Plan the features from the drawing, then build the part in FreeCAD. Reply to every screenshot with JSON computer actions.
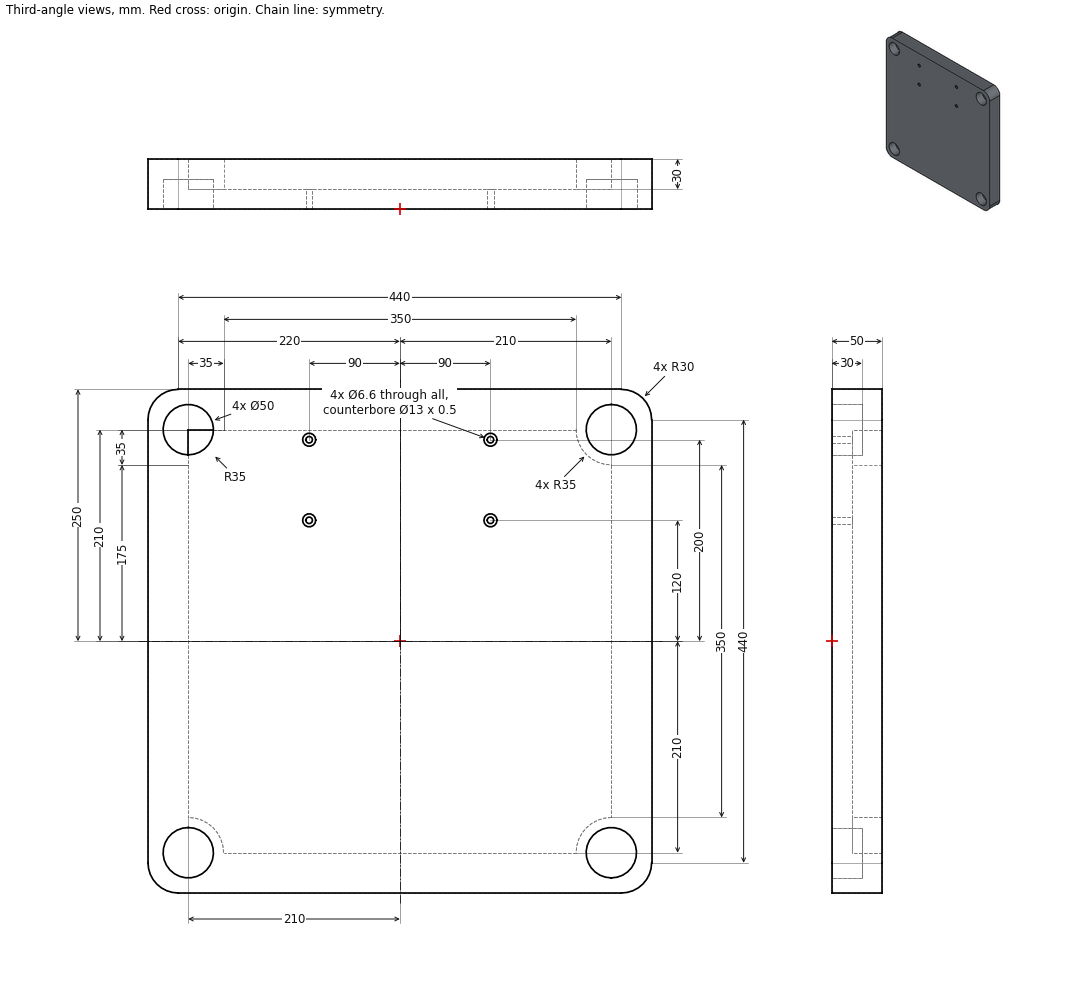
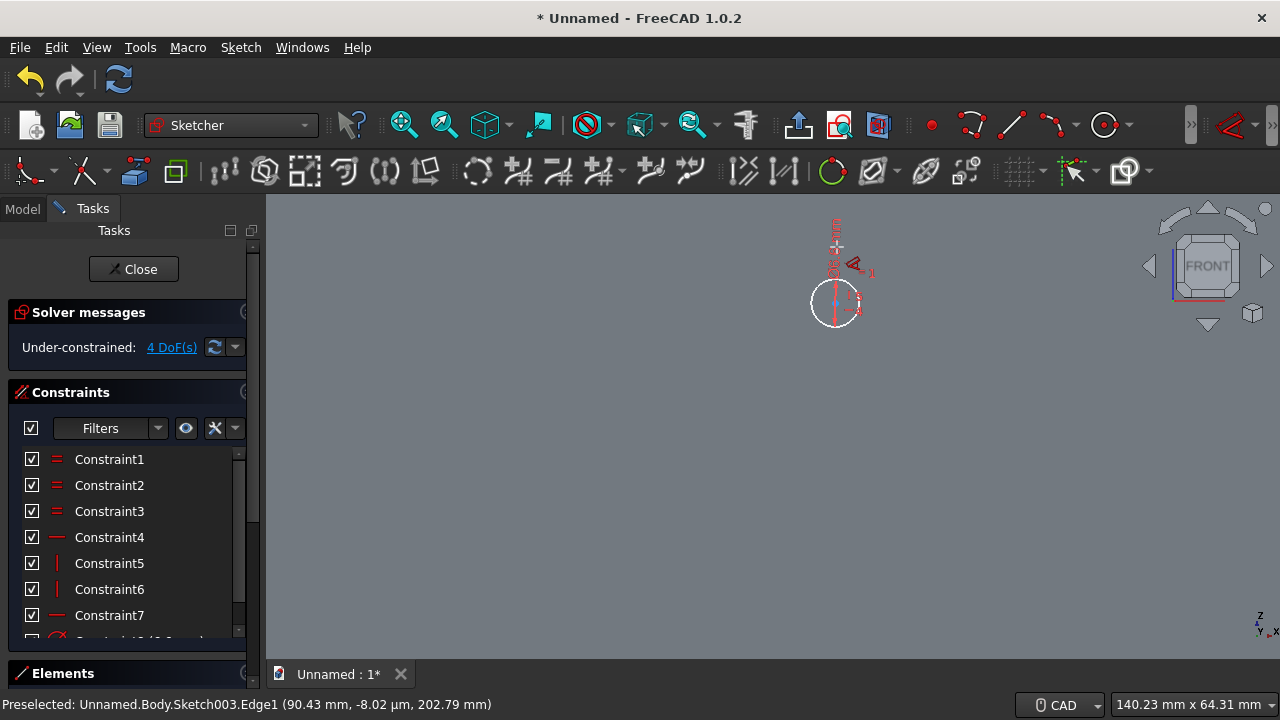
{"action": "scroll", "coordinate": [836, 279], "scroll_direction": "down", "scroll_amount": 8}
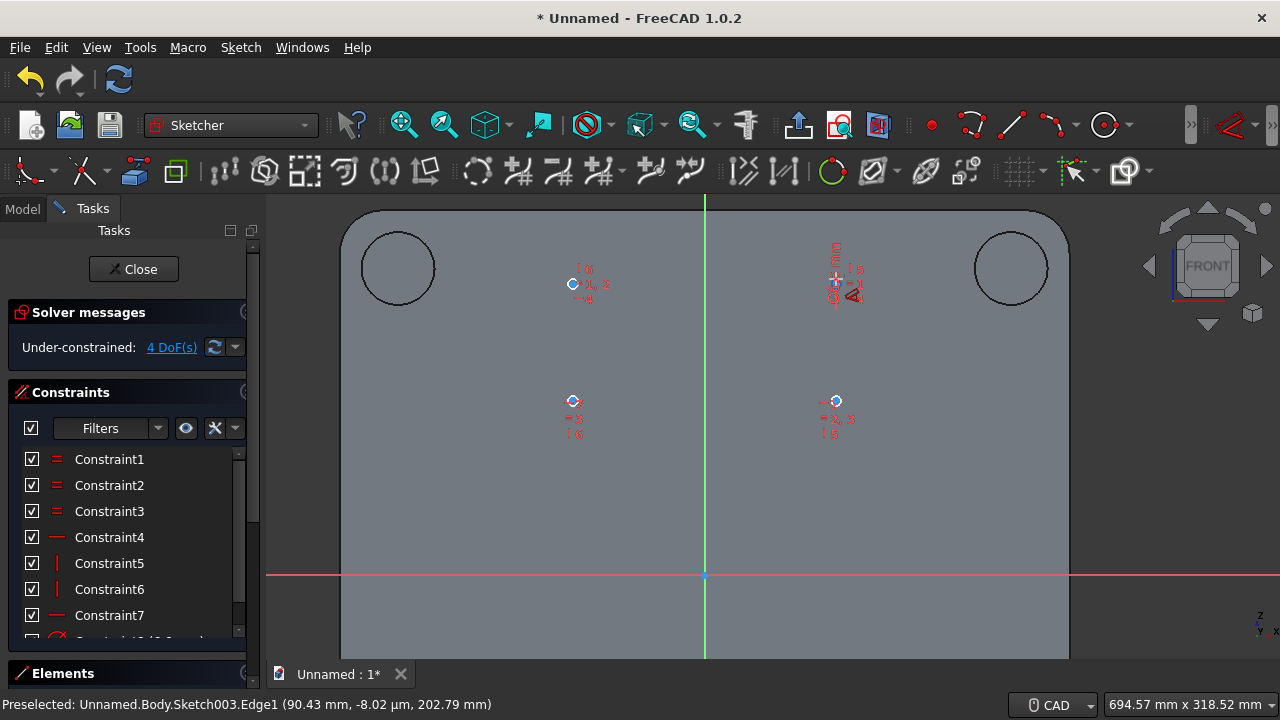
{"action": "left_click", "coordinate": [836, 284]}
{"action": "left_click", "coordinate": [770, 609]}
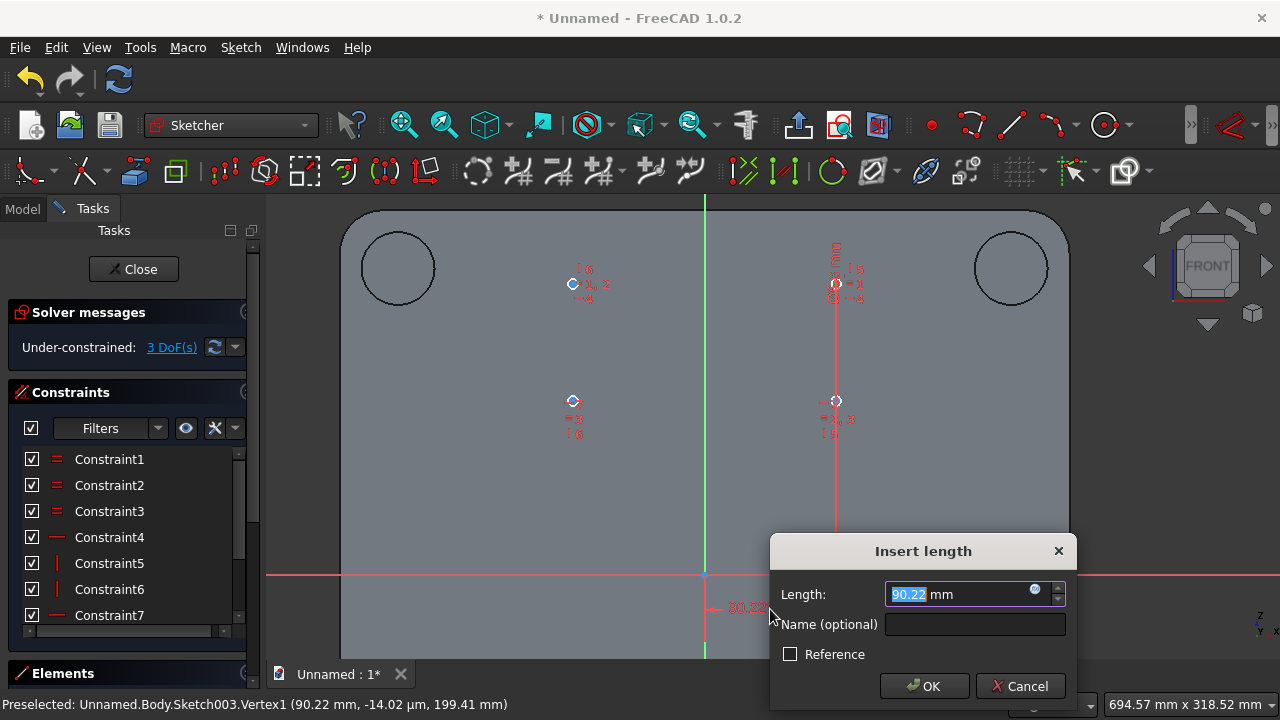
{"action": "type", "text": "90"}
{"action": "key", "text": "Return"}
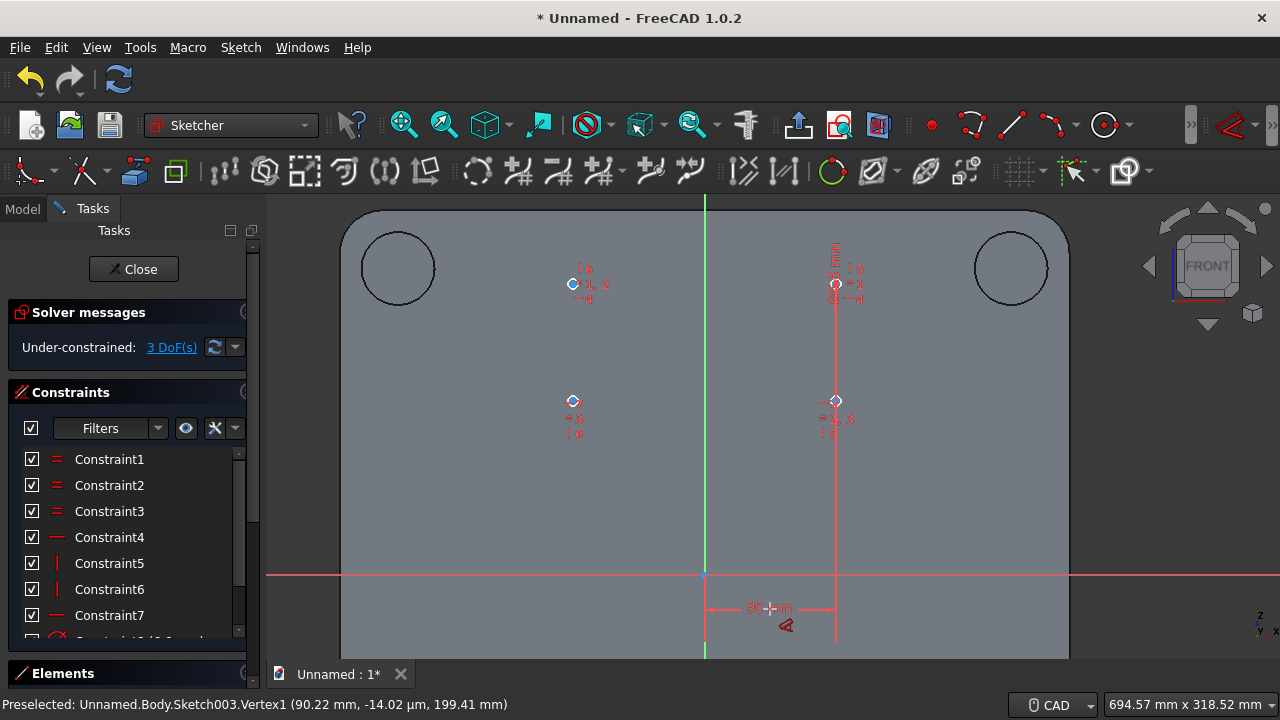
{"action": "left_click", "coordinate": [573, 284]}
{"action": "left_click", "coordinate": [639, 609]}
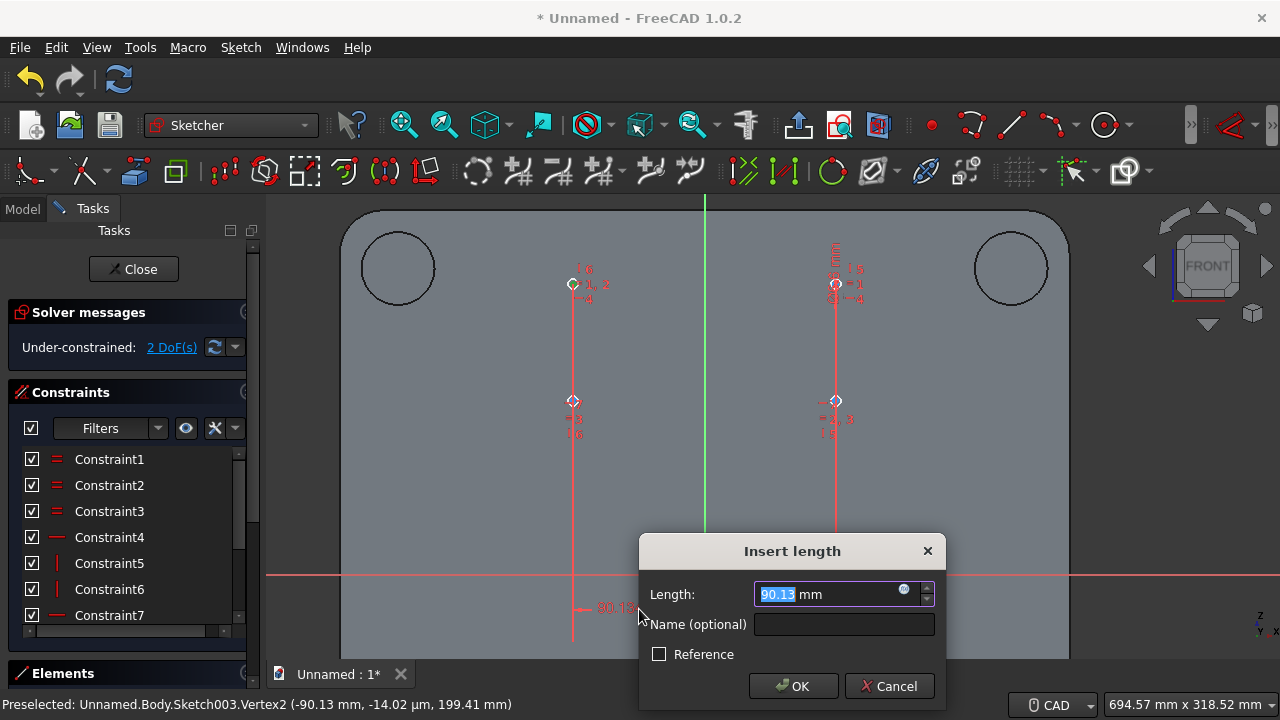
{"action": "type", "text": "90"}
{"action": "key", "text": "Return"}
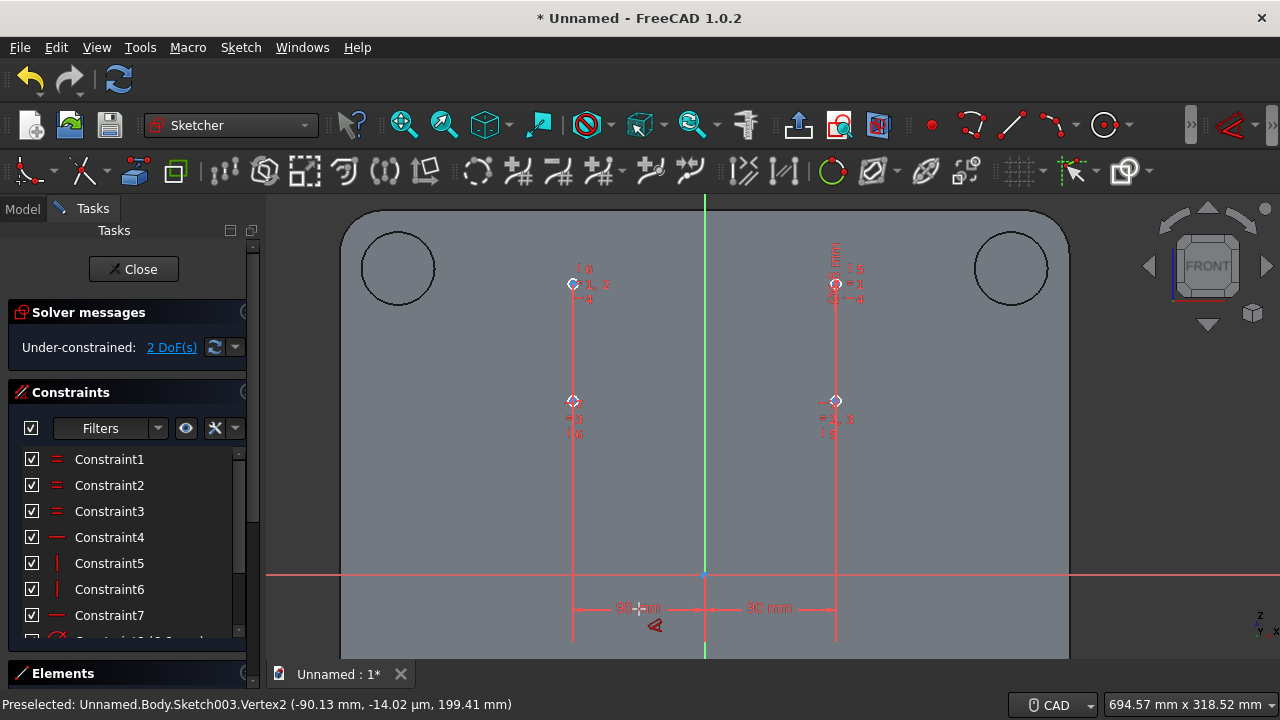
{"action": "left_click", "coordinate": [836, 284]}
{"action": "left_click", "coordinate": [870, 430]}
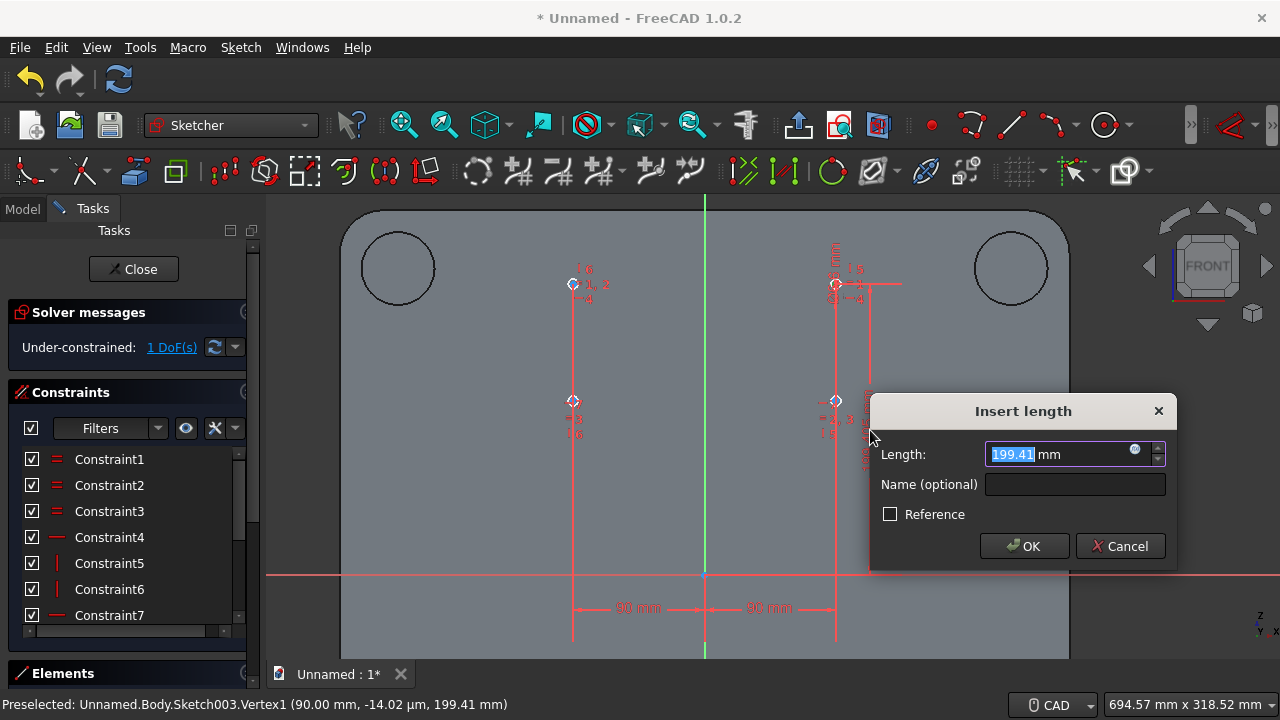
{"action": "type", "text": "200"}
{"action": "key", "text": "Return"}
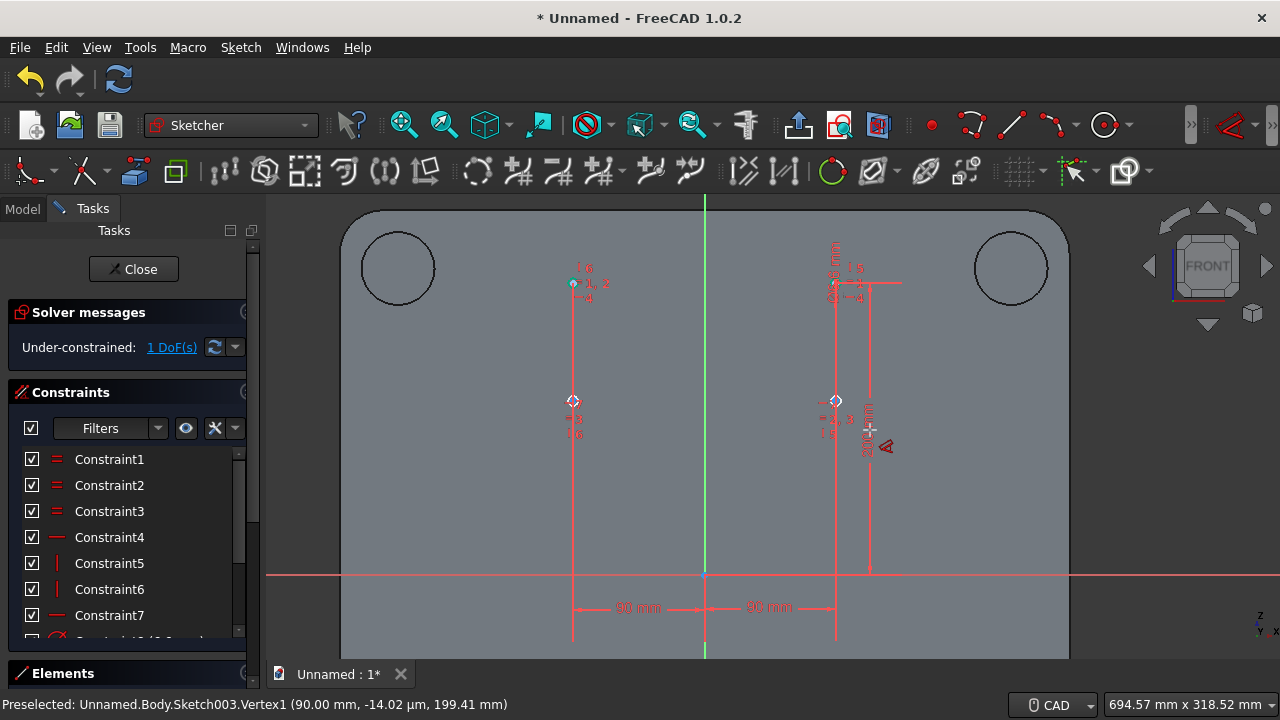
{"action": "left_click", "coordinate": [836, 401]}
{"action": "left_click", "coordinate": [870, 488]}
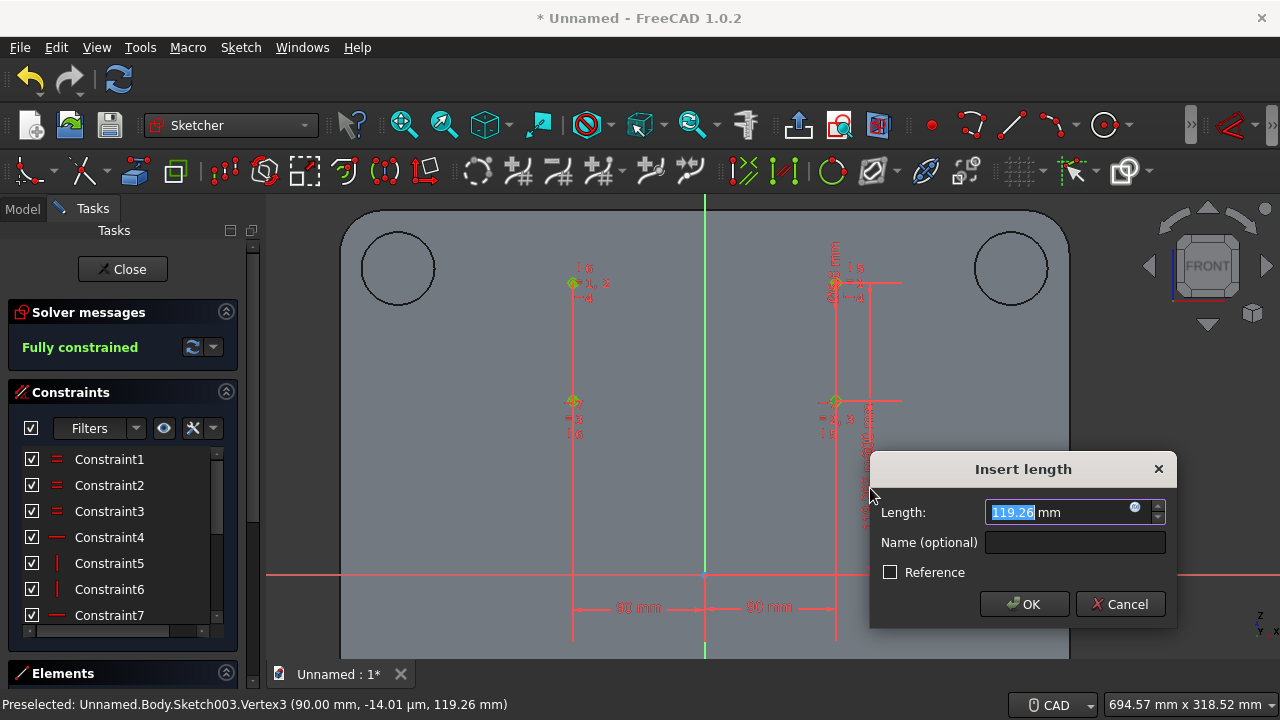
{"action": "type", "text": "120"}
{"action": "key", "text": "Return"}
{"action": "key", "text": "Escape"}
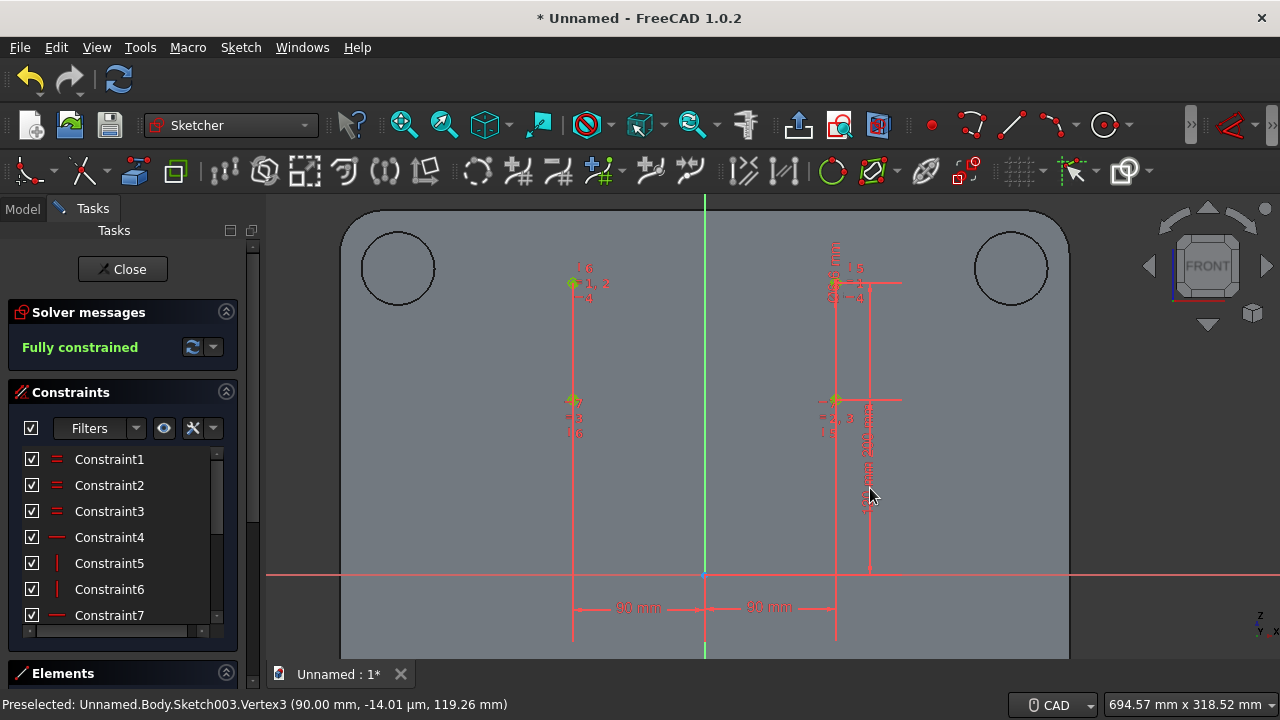
{"action": "left_click", "coordinate": [123, 269]}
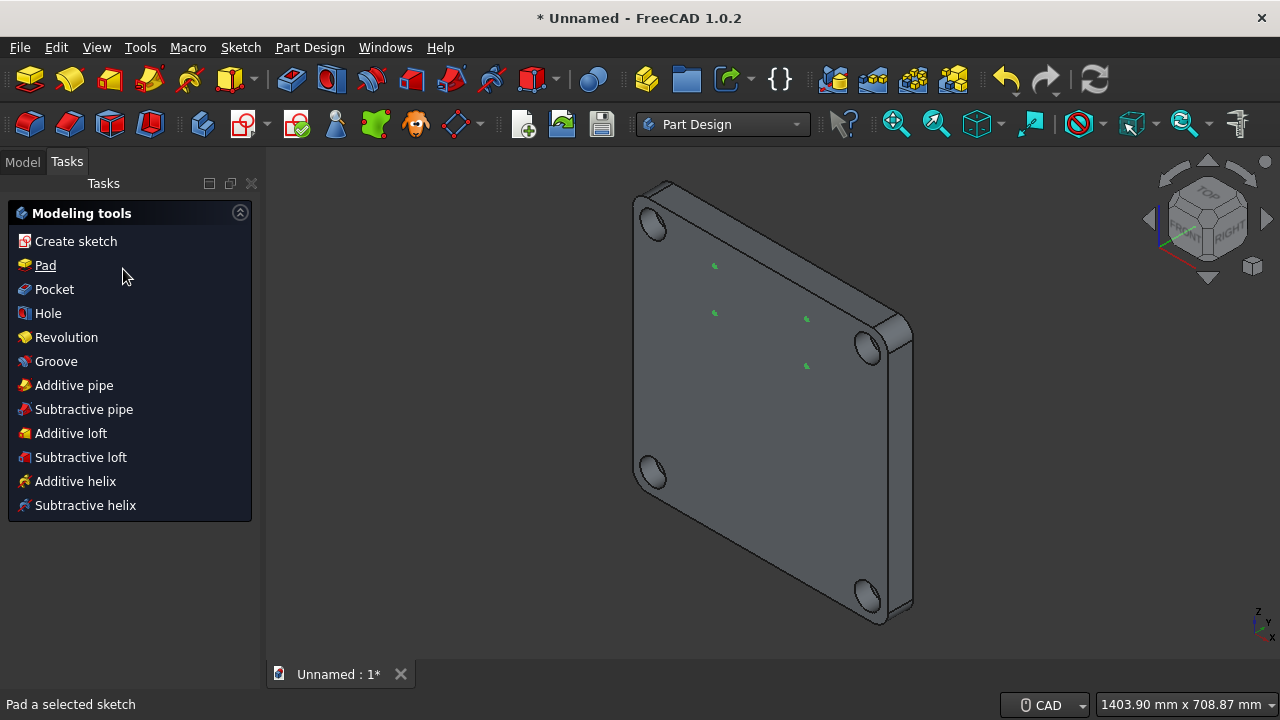
{"action": "left_click", "coordinate": [332, 80]}